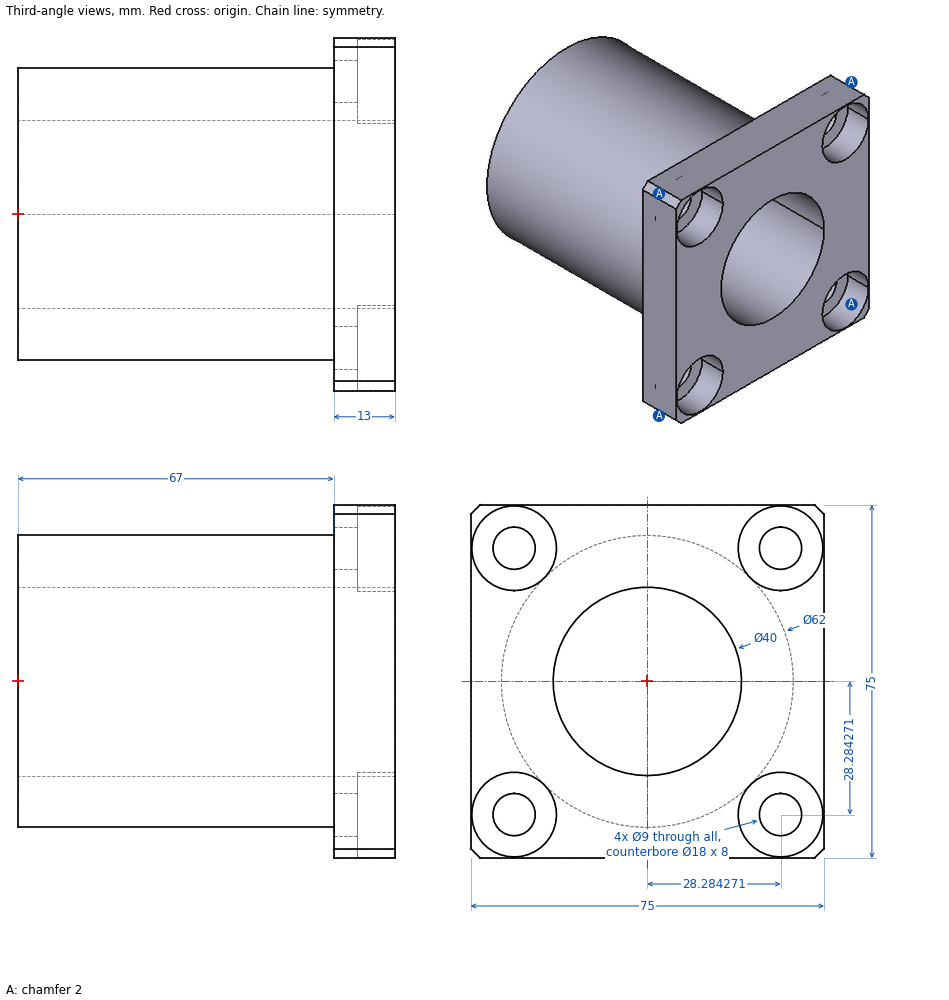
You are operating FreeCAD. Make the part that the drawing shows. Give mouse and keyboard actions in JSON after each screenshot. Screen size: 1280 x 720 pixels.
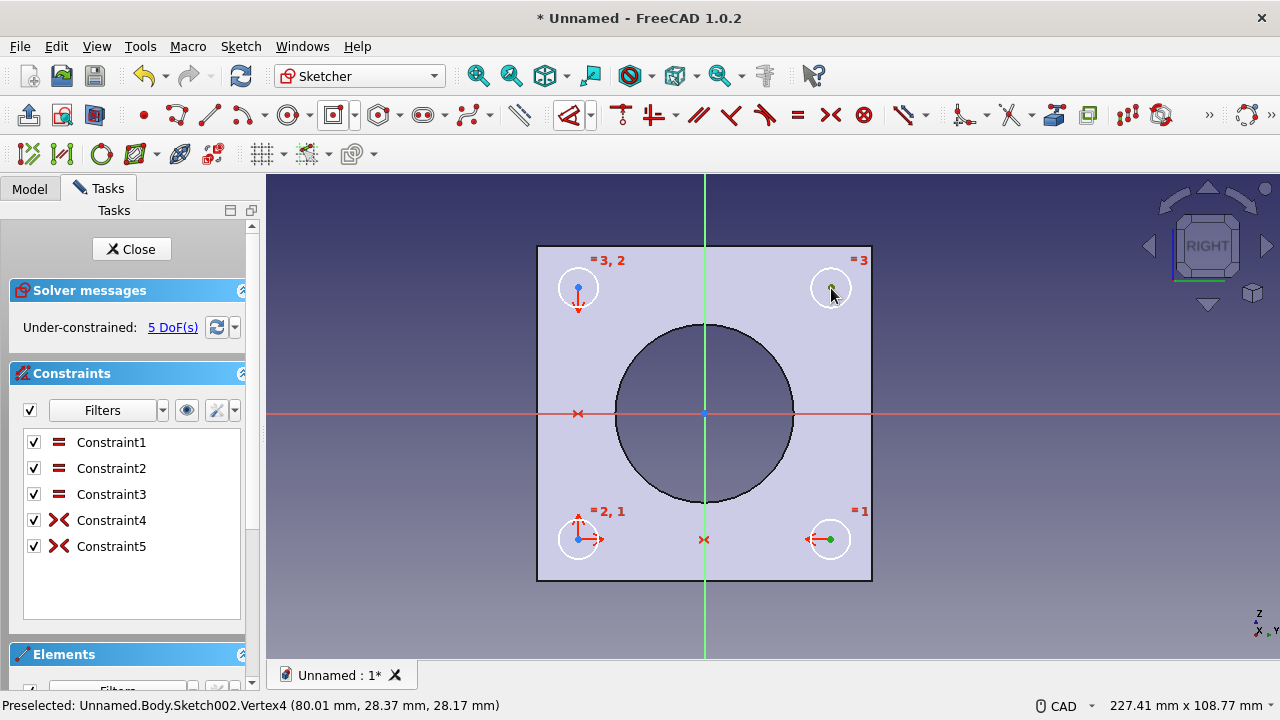
{"action": "left_click", "coordinate": [353, 414]}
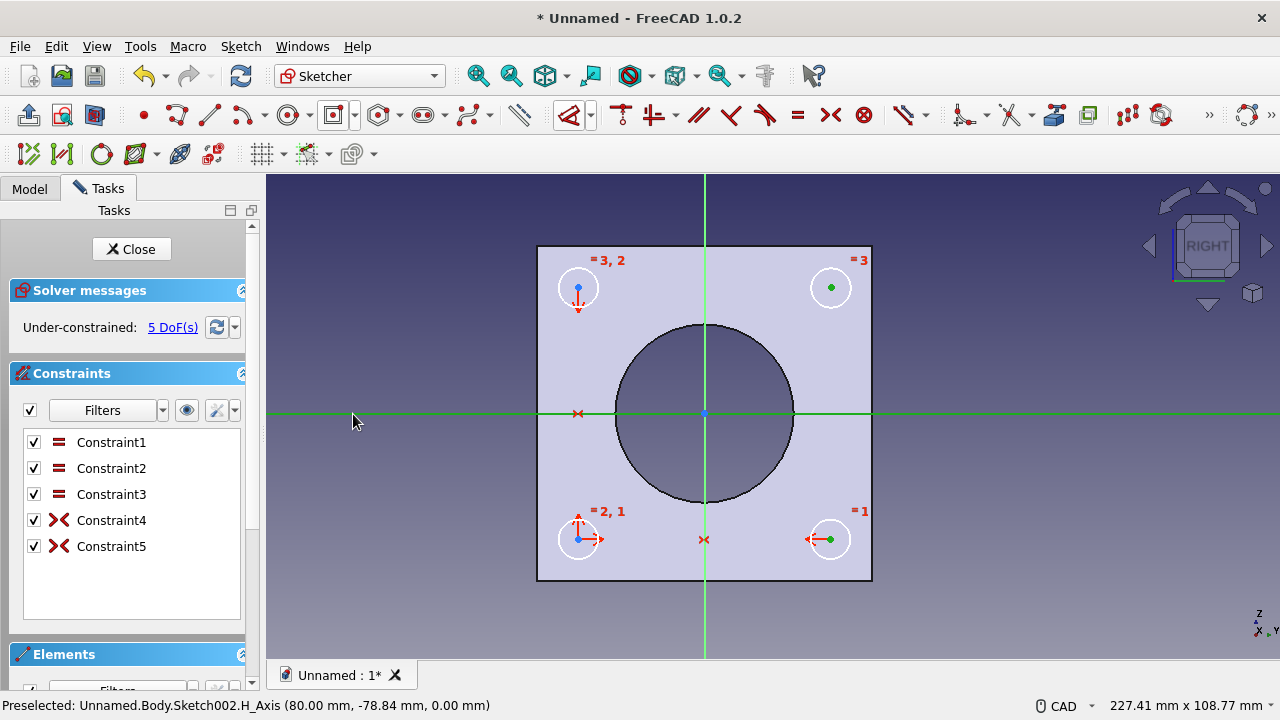
{"action": "left_click", "coordinate": [831, 116]}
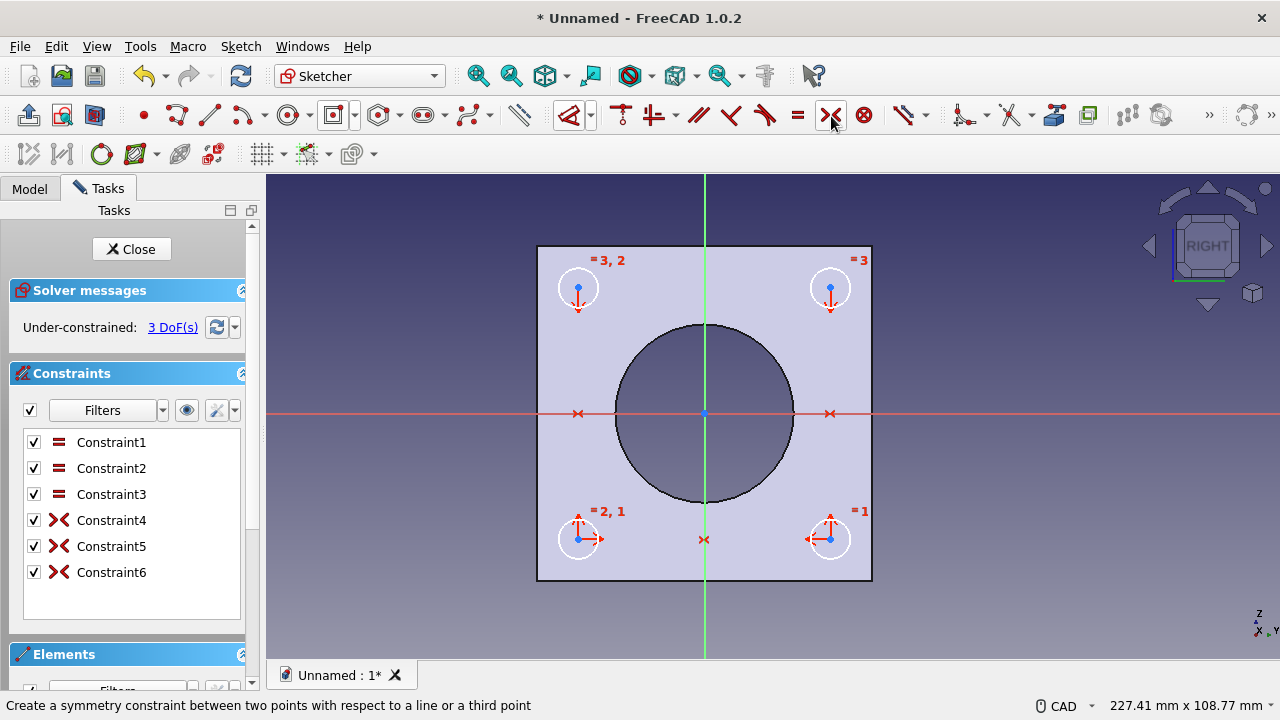
{"action": "left_click", "coordinate": [844, 525]}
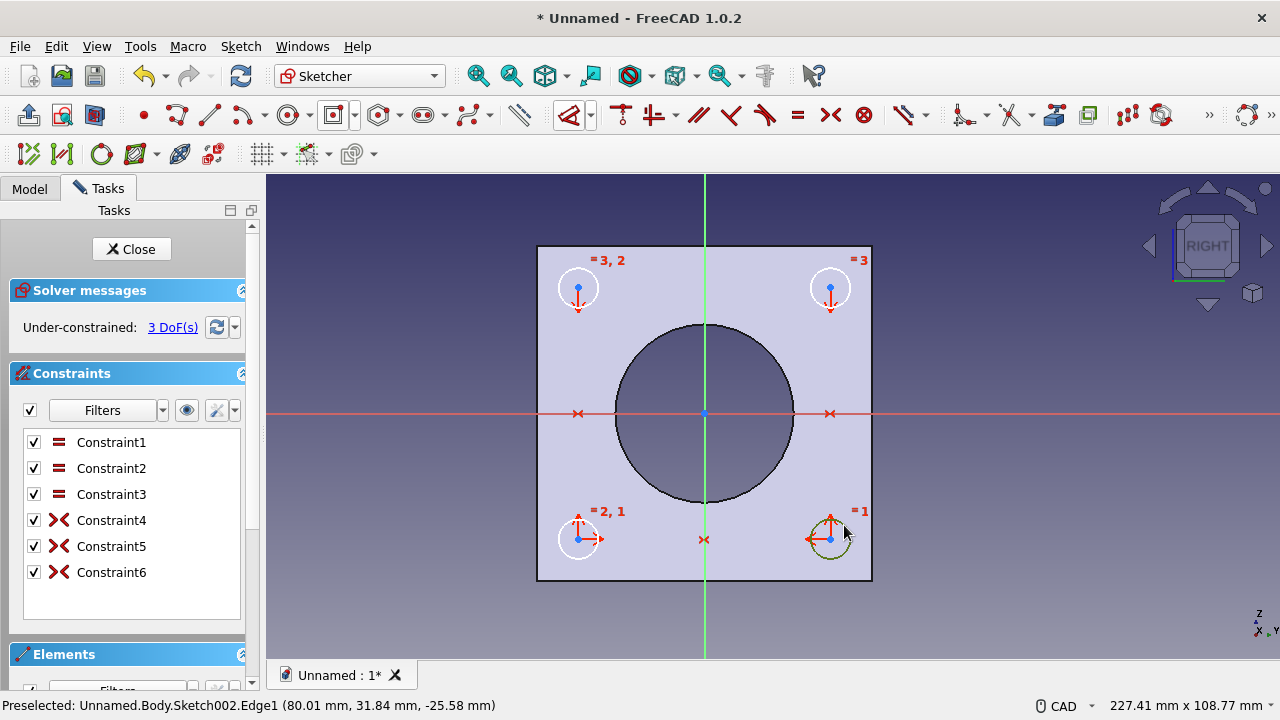
{"action": "left_click", "coordinate": [590, 116]}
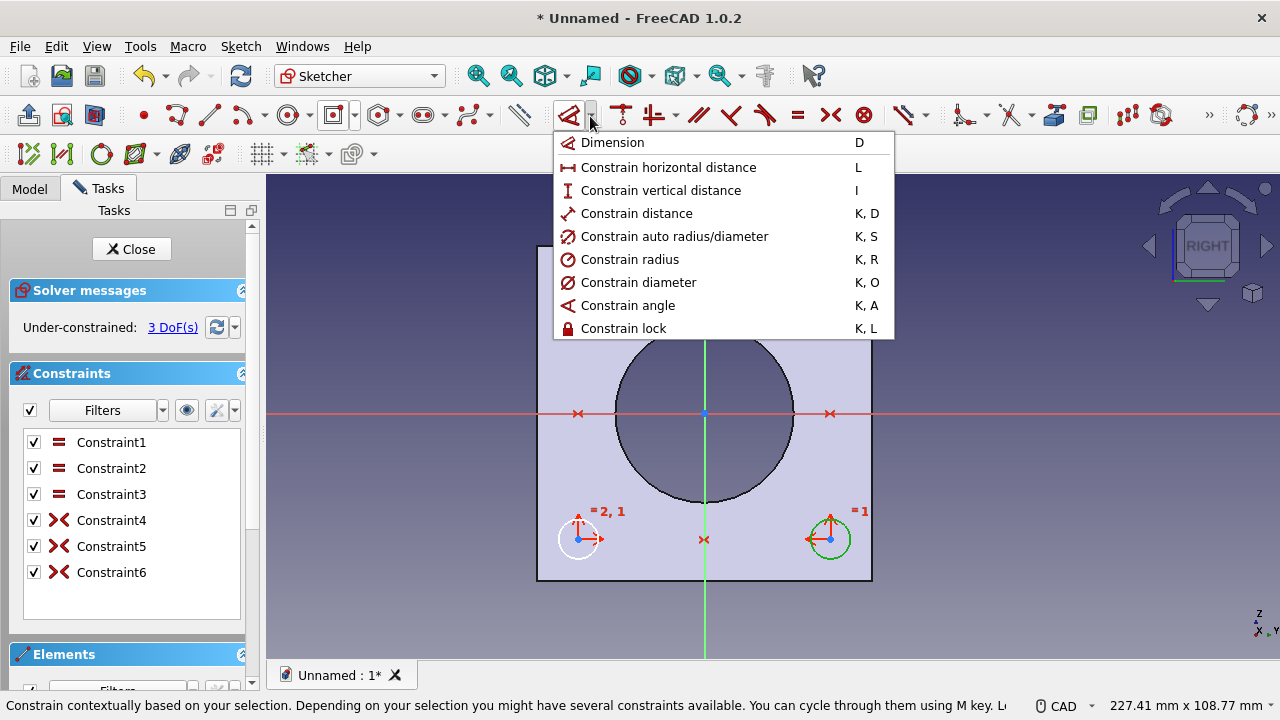
{"action": "left_click", "coordinate": [724, 282]}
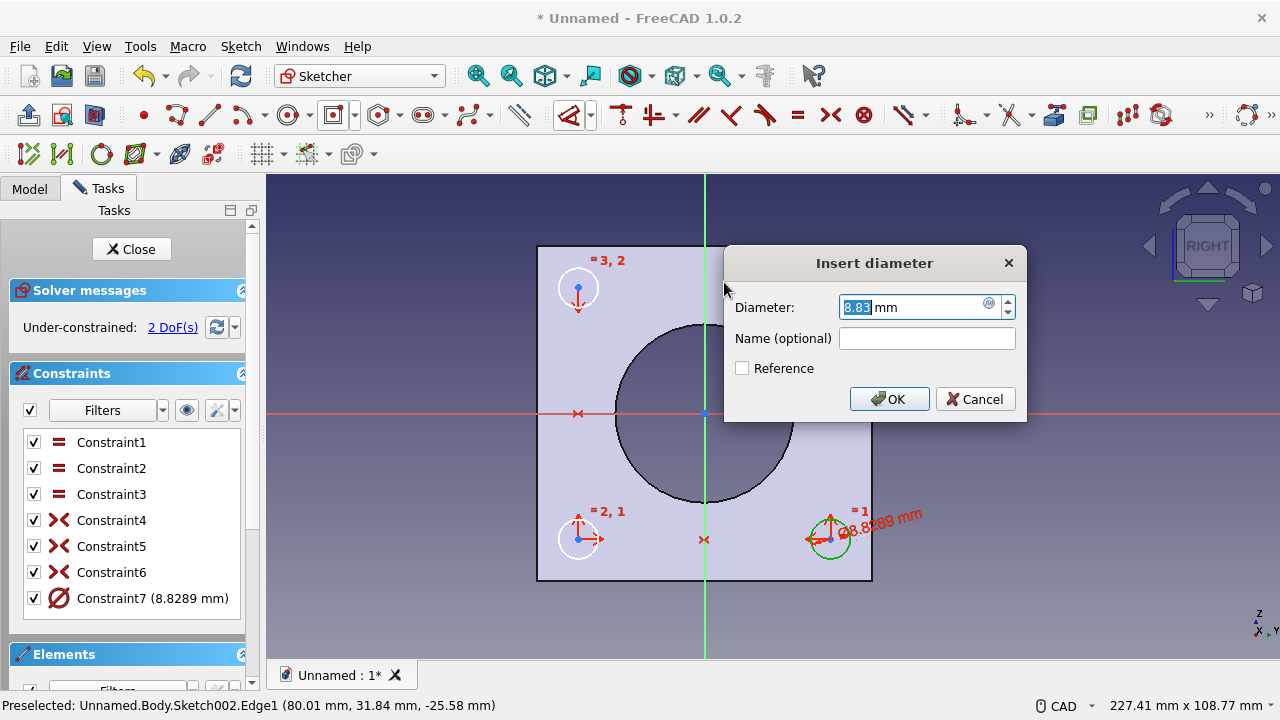
{"action": "type", "text": "9"}
{"action": "key", "text": "Return"}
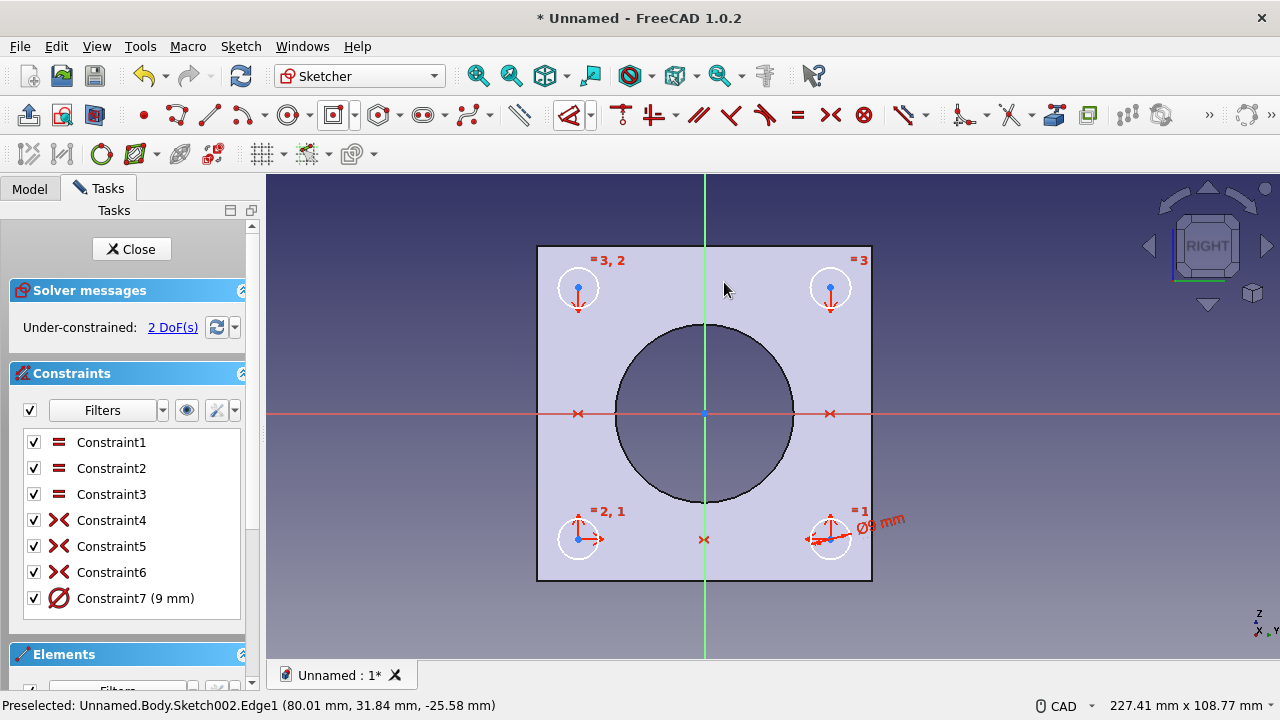
{"action": "left_click", "coordinate": [831, 539]}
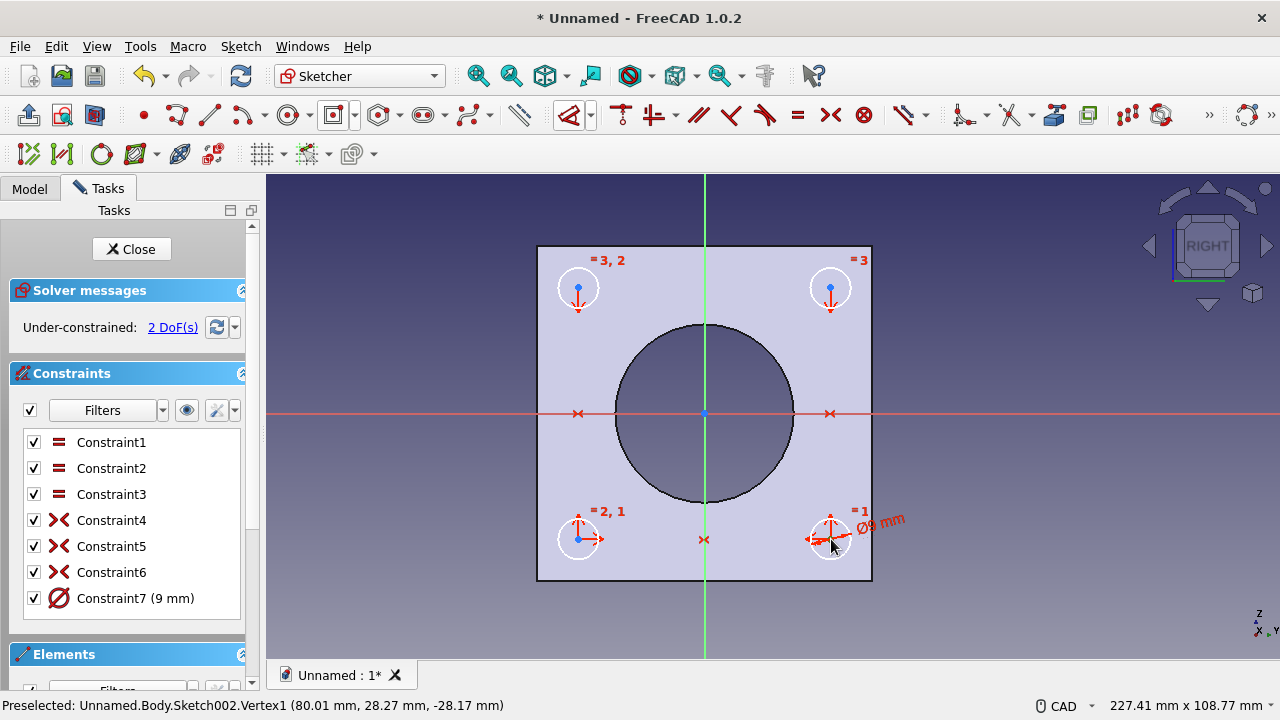
{"action": "left_click", "coordinate": [590, 116]}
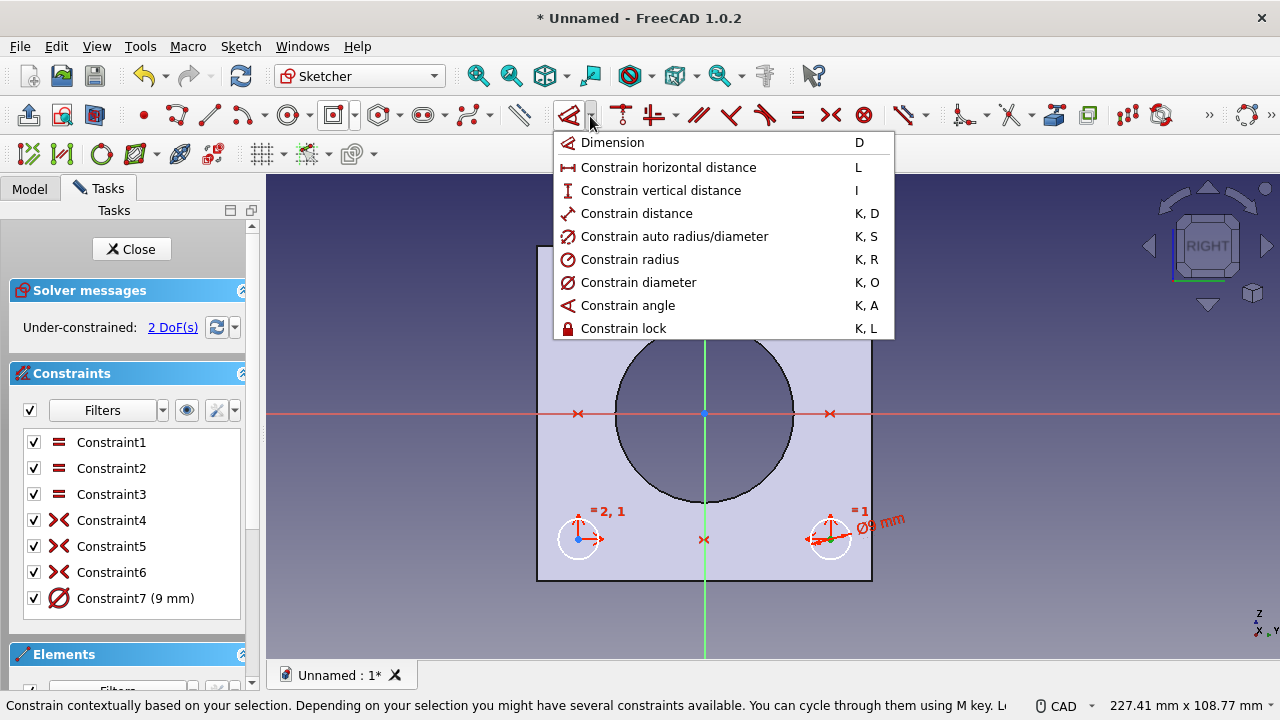
{"action": "left_click", "coordinate": [724, 168]}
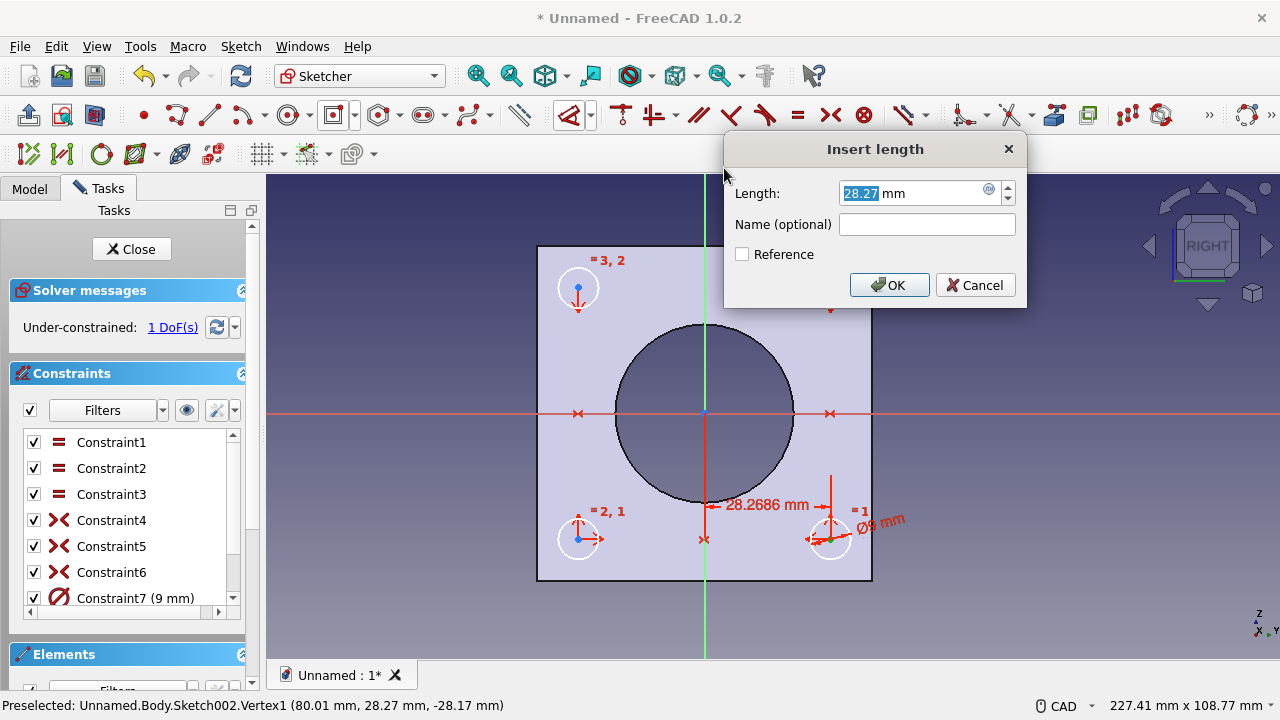
{"action": "type", "text": "28.284271"}
{"action": "key", "text": "Return"}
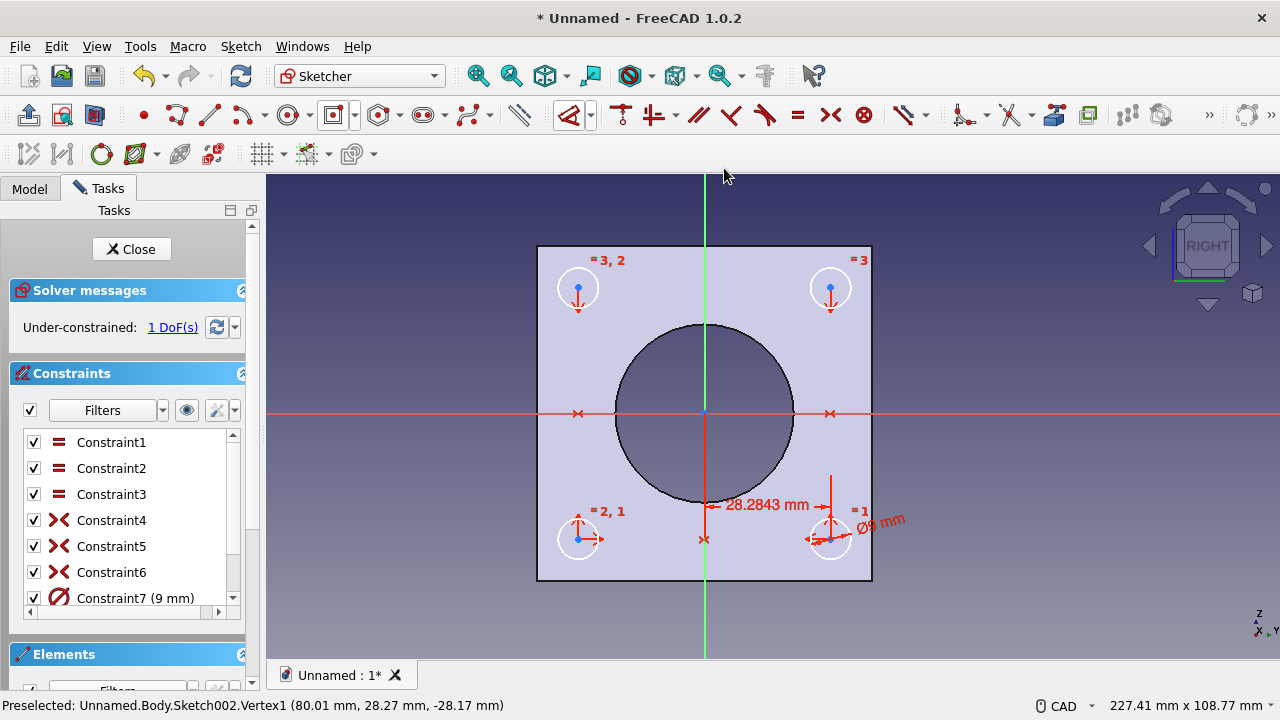
{"action": "left_click", "coordinate": [831, 539]}